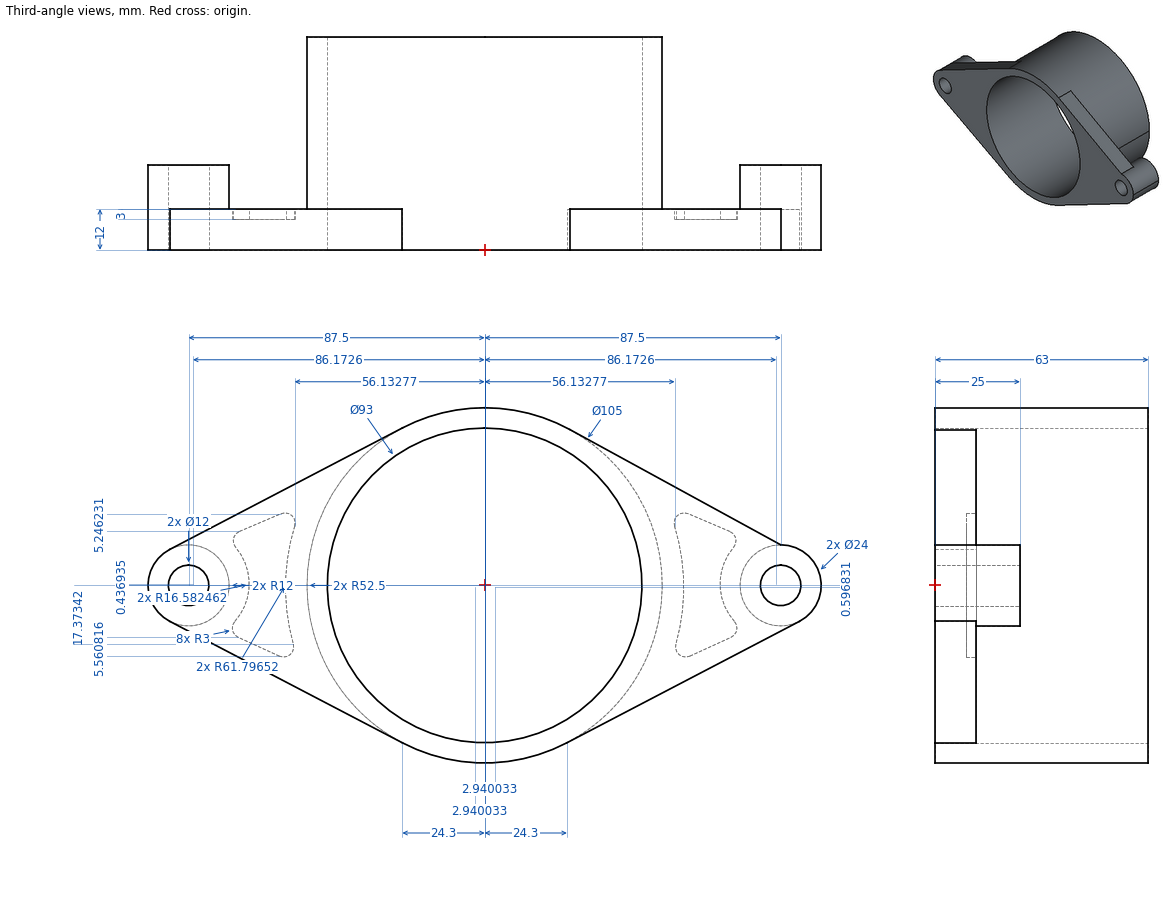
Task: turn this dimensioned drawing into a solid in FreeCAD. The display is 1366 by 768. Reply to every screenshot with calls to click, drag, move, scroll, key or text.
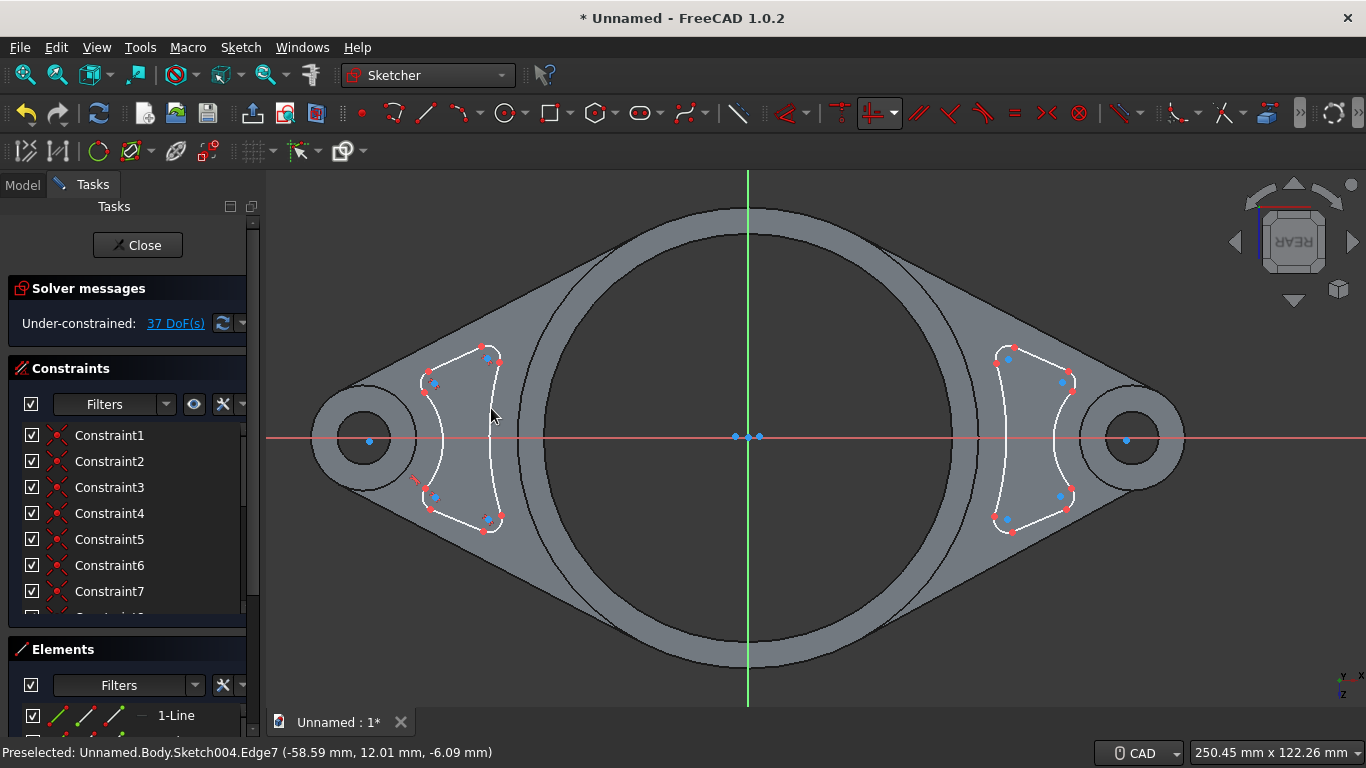
click(491, 408)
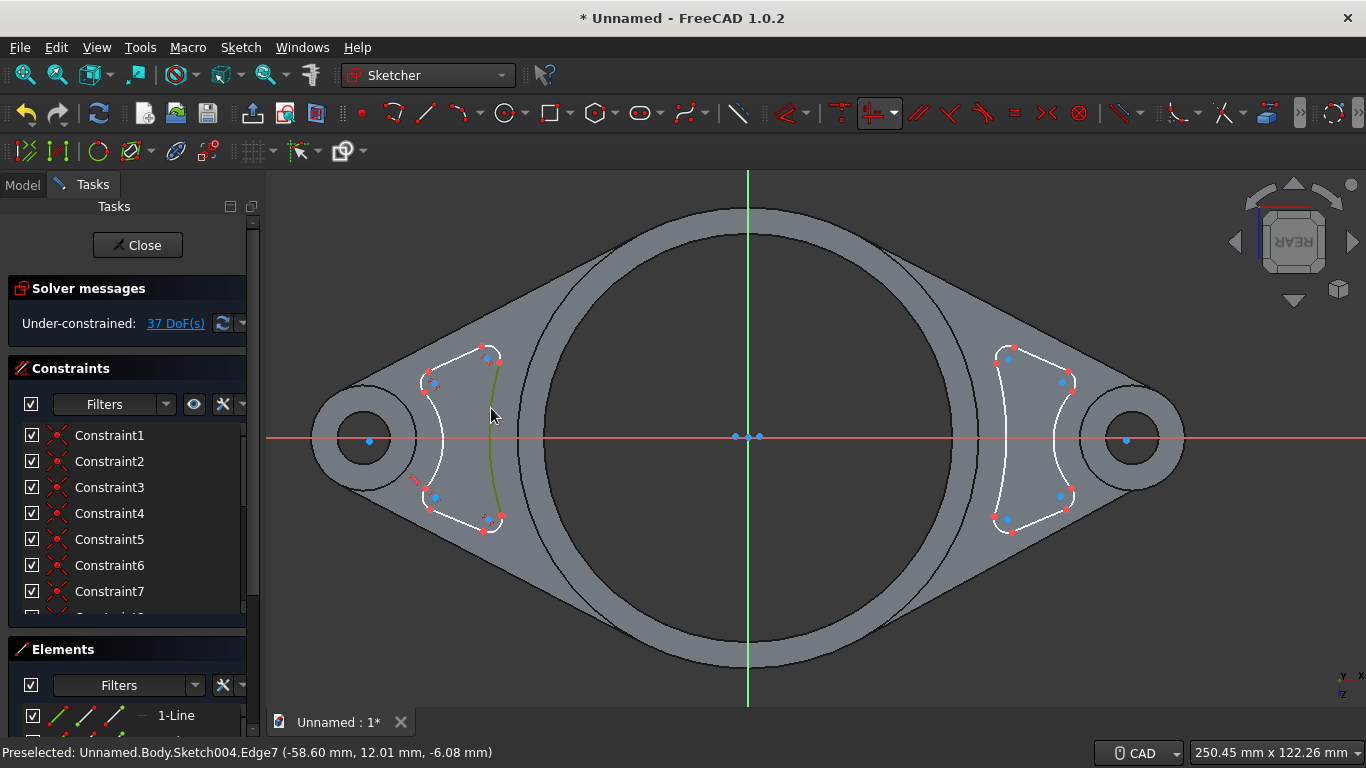
click(496, 349)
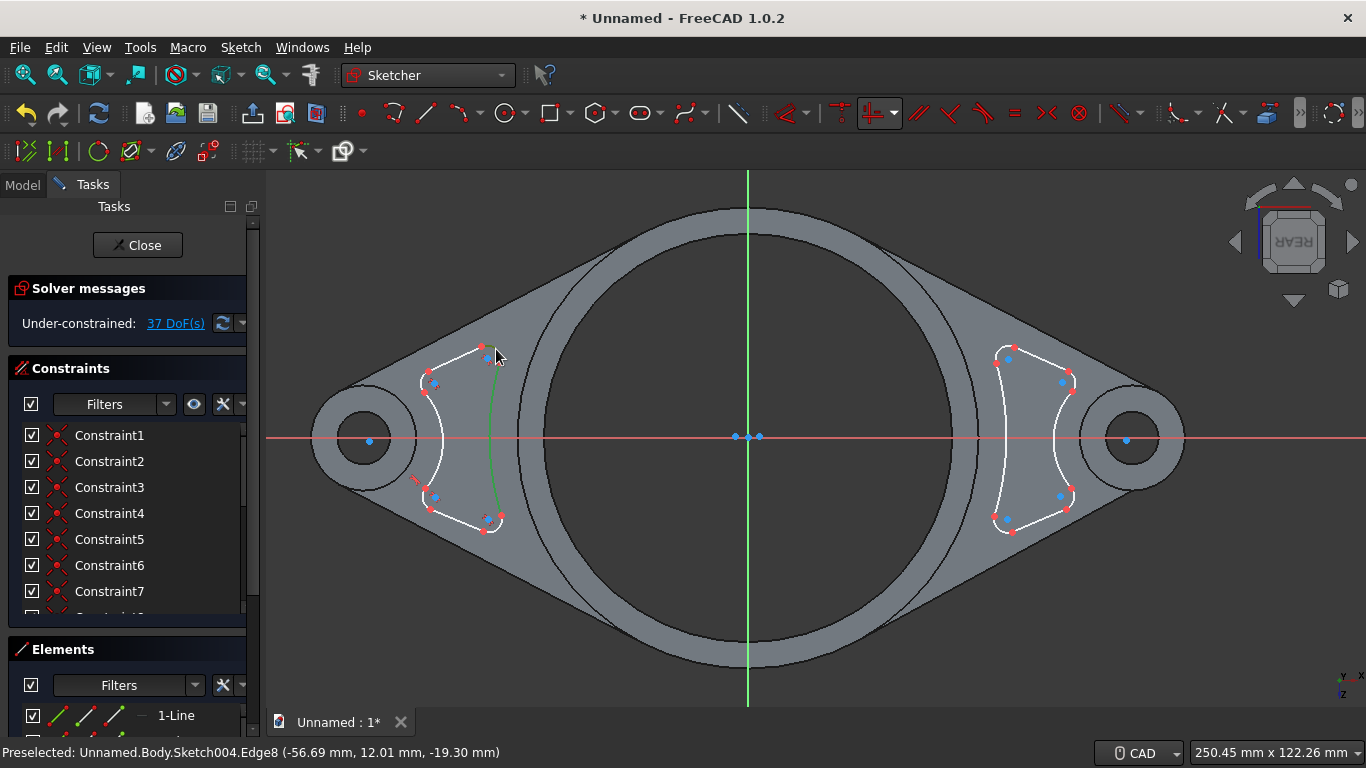
click(984, 114)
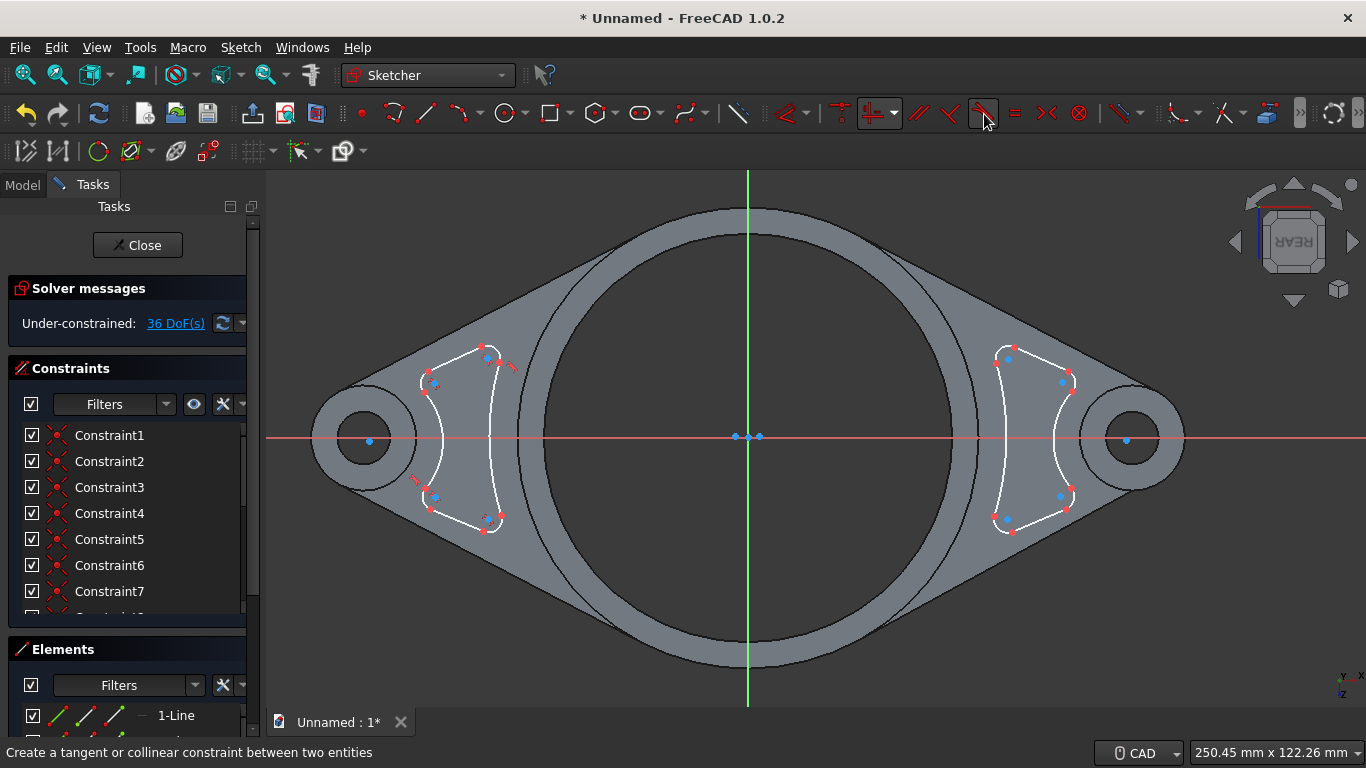
click(1052, 364)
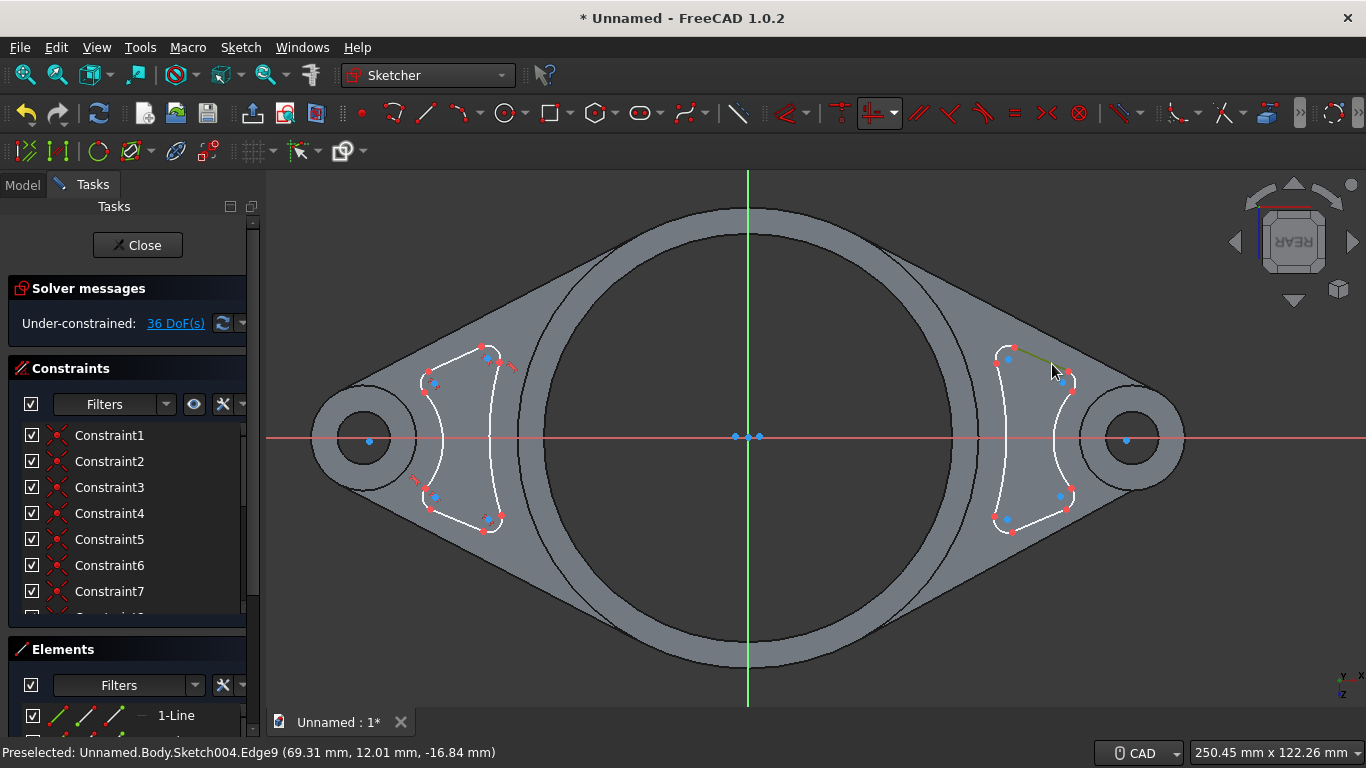
click(1000, 349)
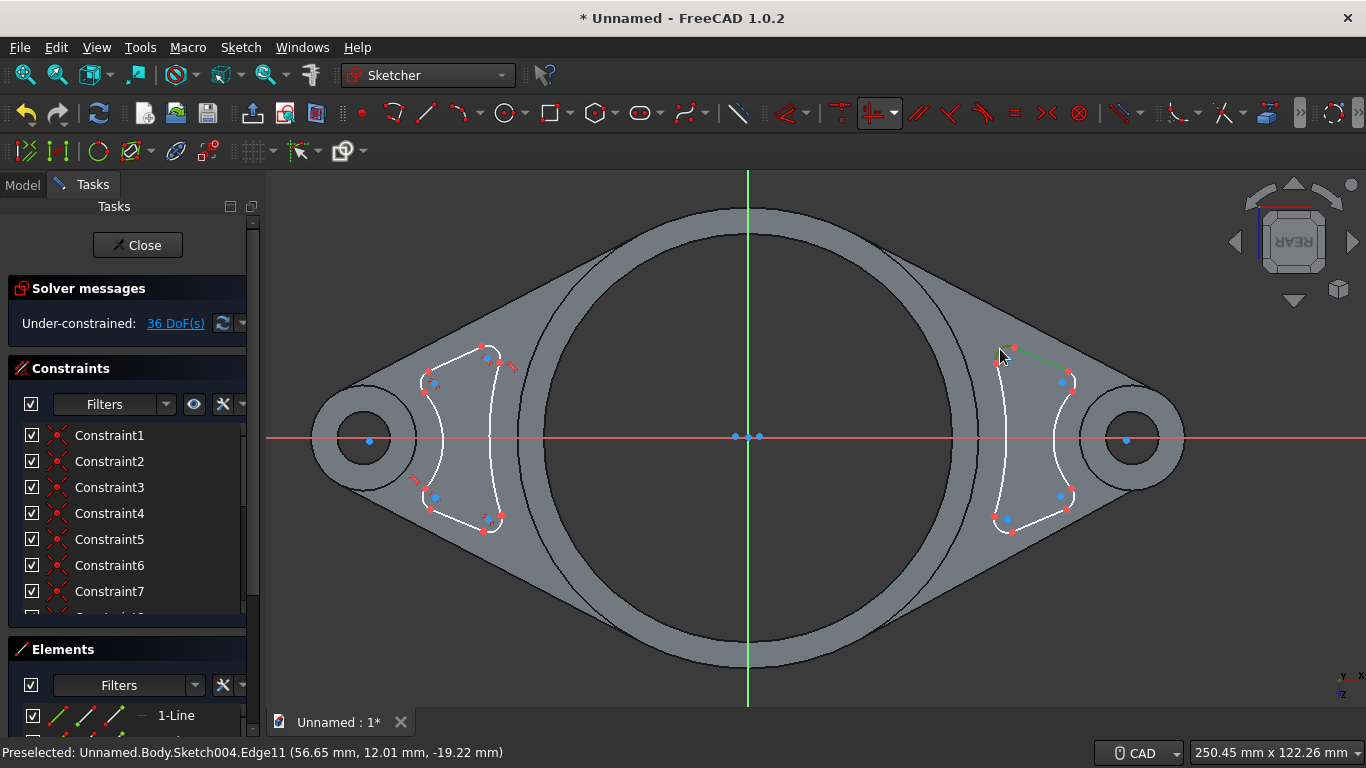
key(t)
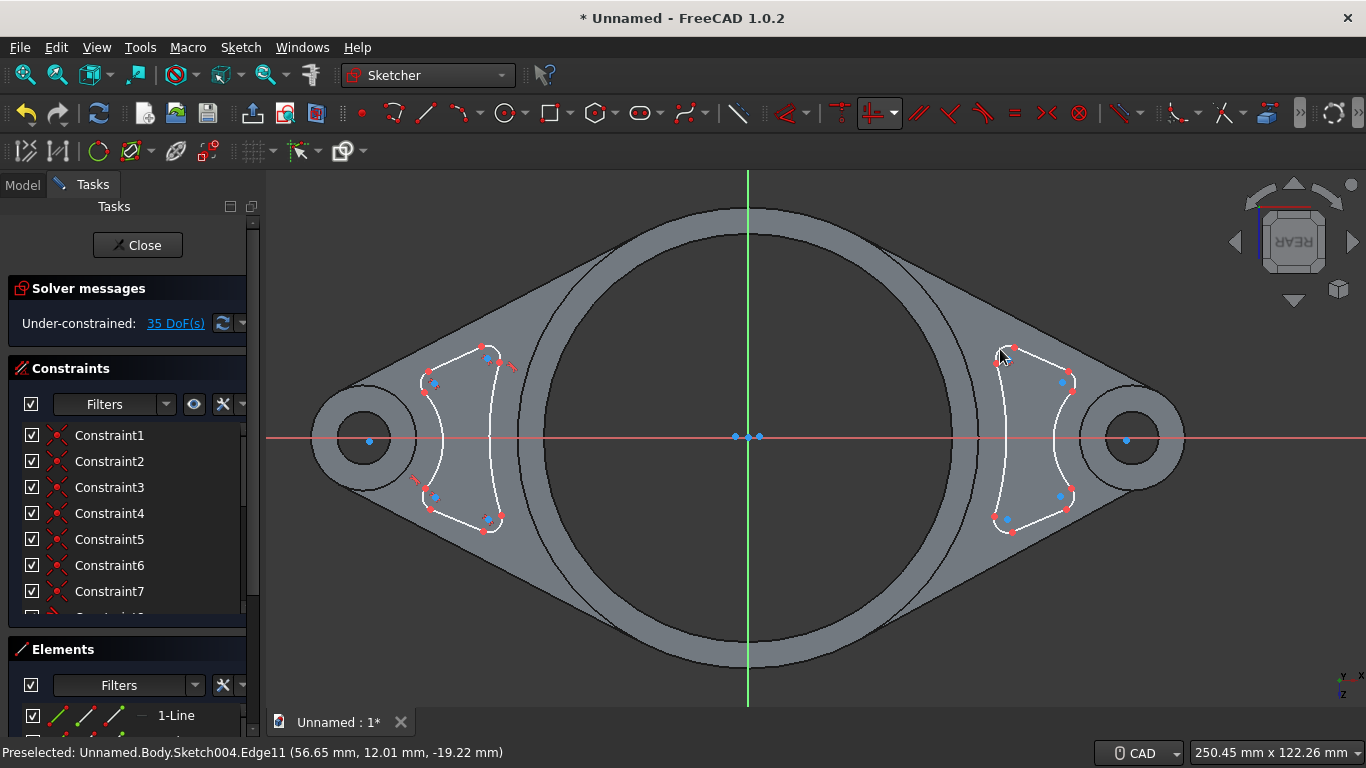
click(1052, 364)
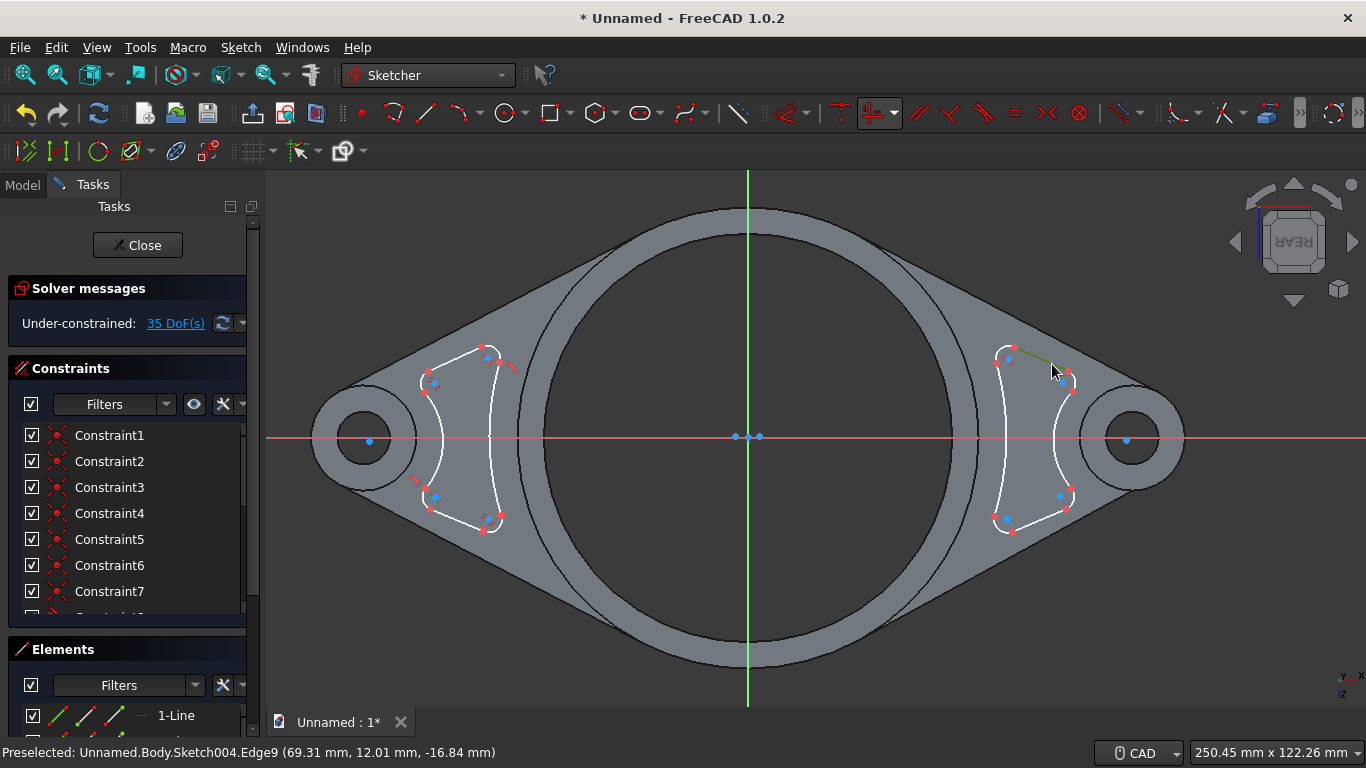
click(1075, 380)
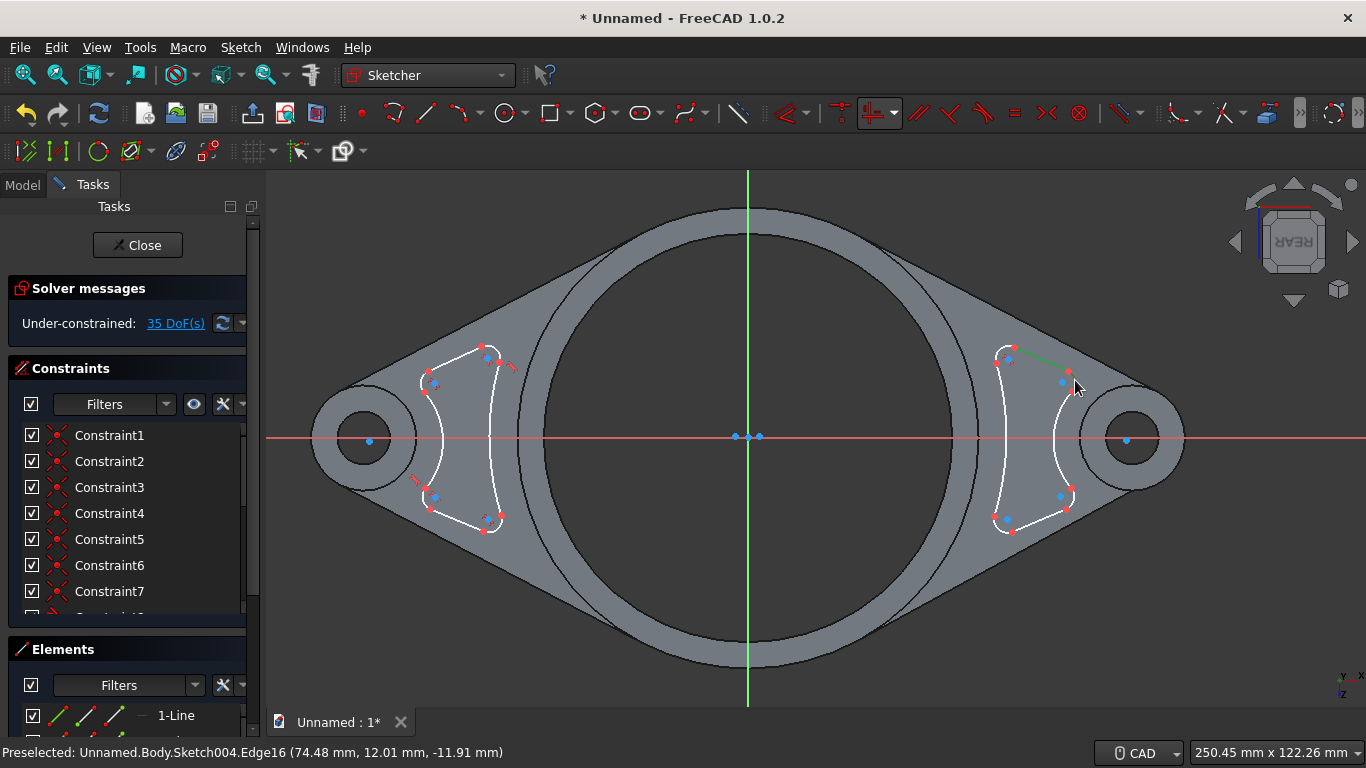
key(t)